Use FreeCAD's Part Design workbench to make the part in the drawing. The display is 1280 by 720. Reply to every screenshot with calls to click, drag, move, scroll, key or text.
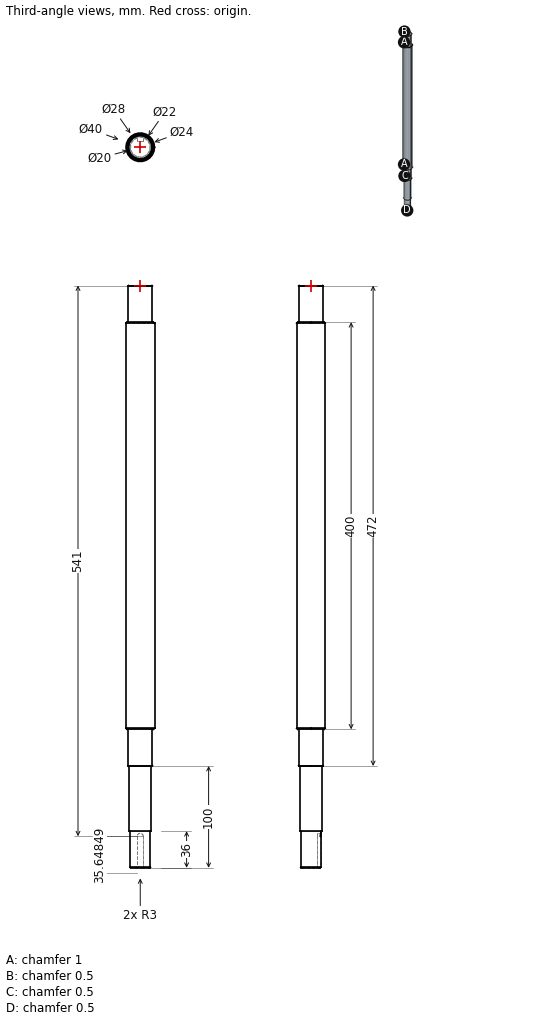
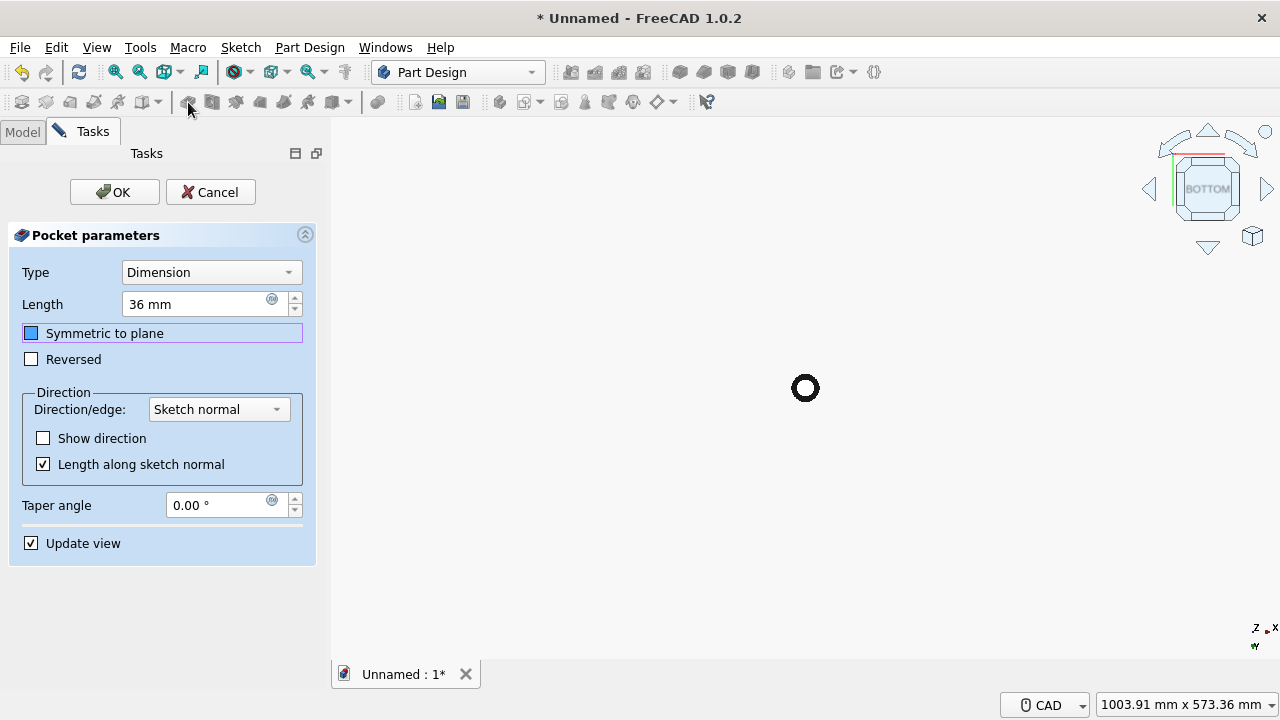
click(115, 192)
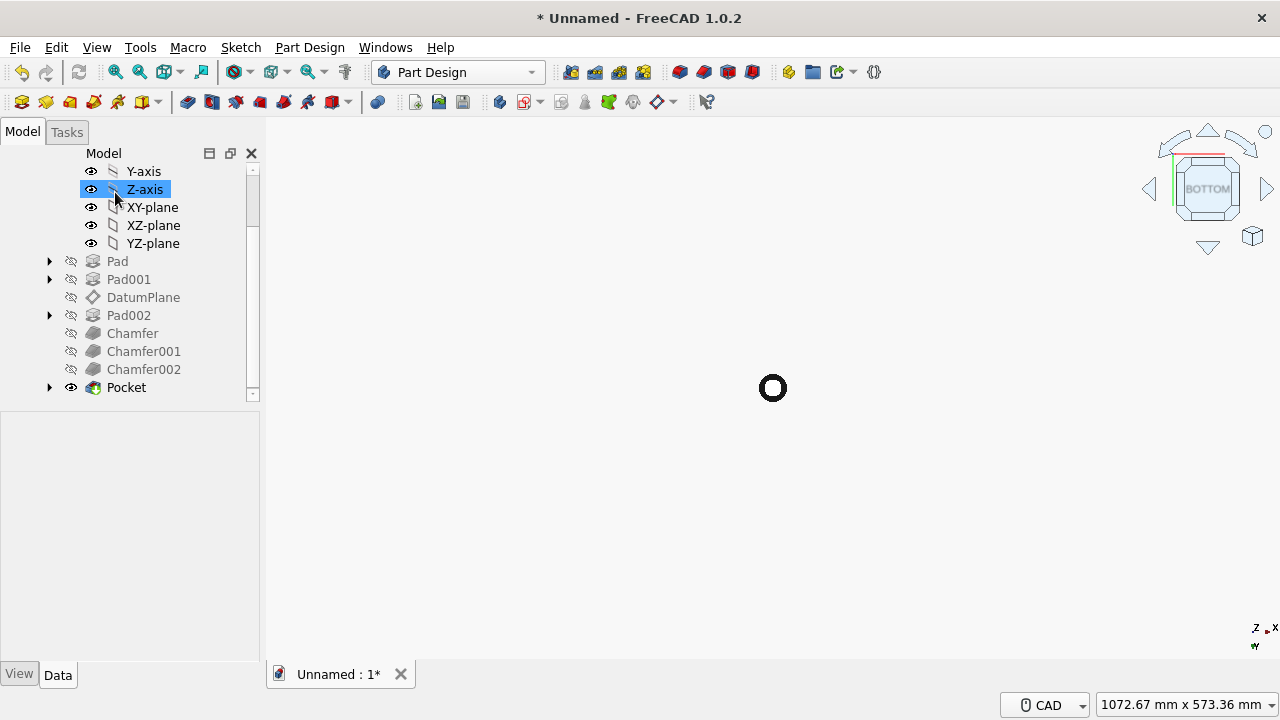
key(v)
key(f)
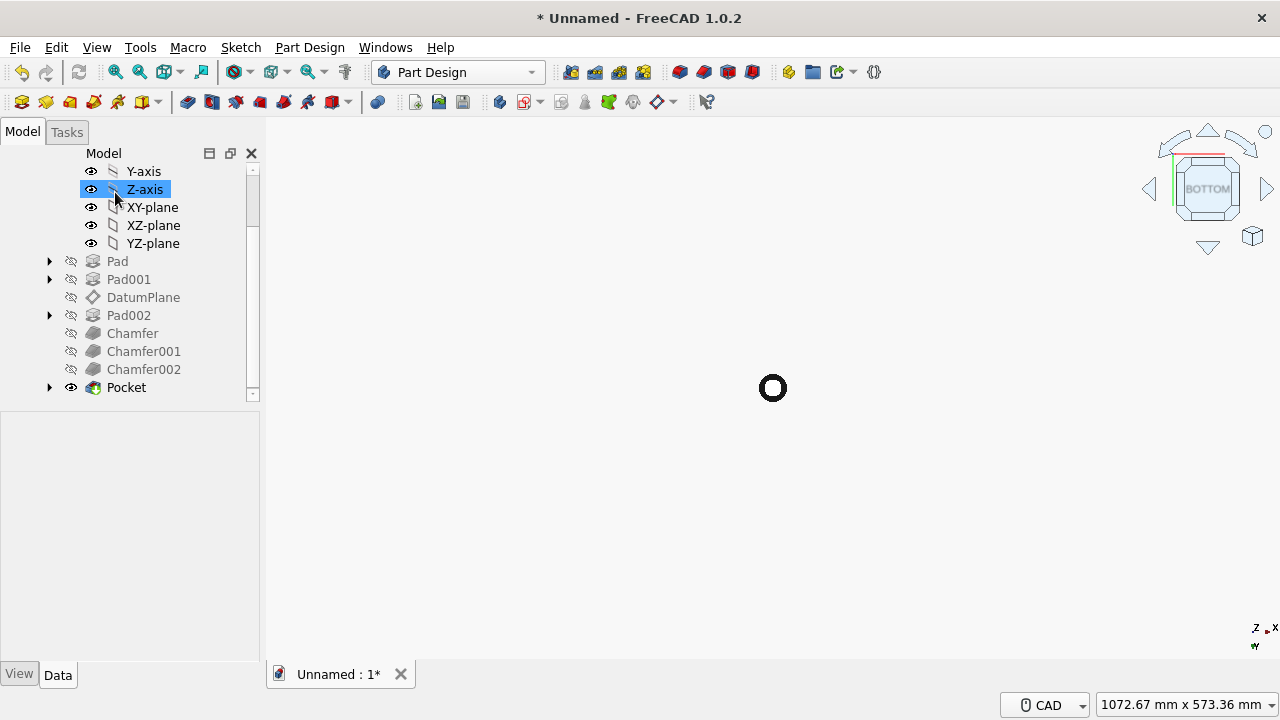
scroll(160, 275, down, 3)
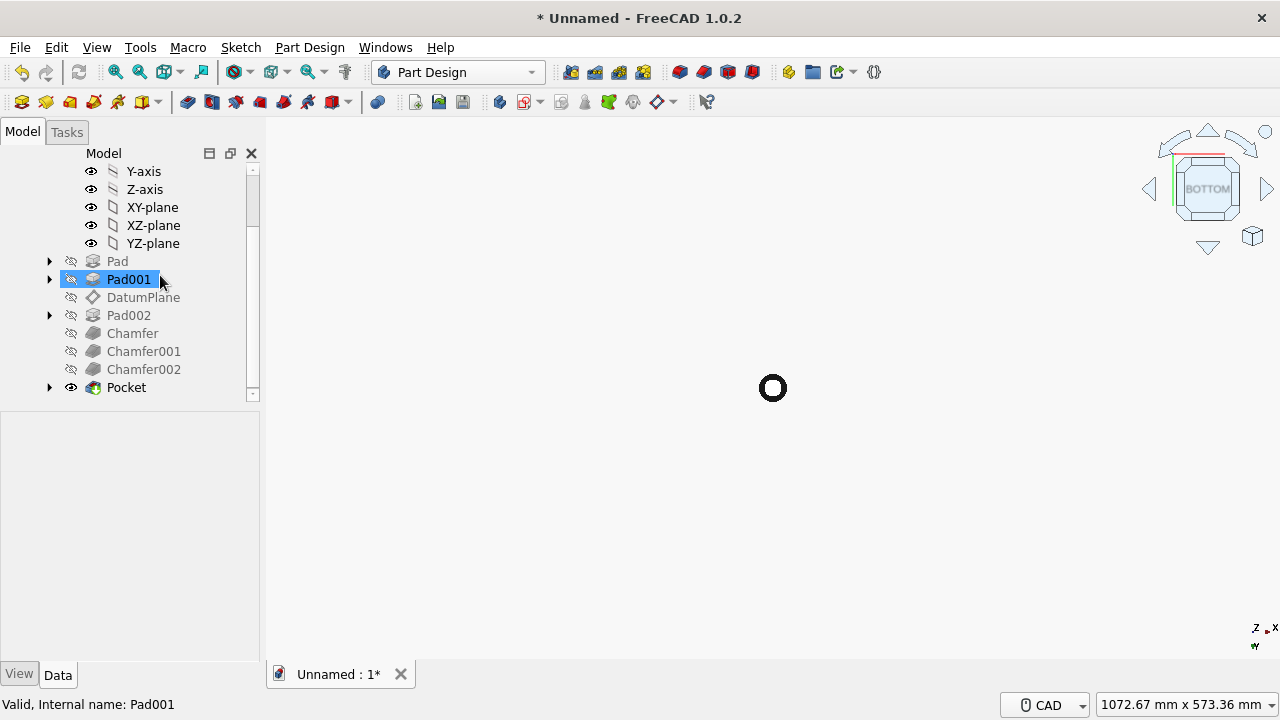
scroll(160, 275, up, 15)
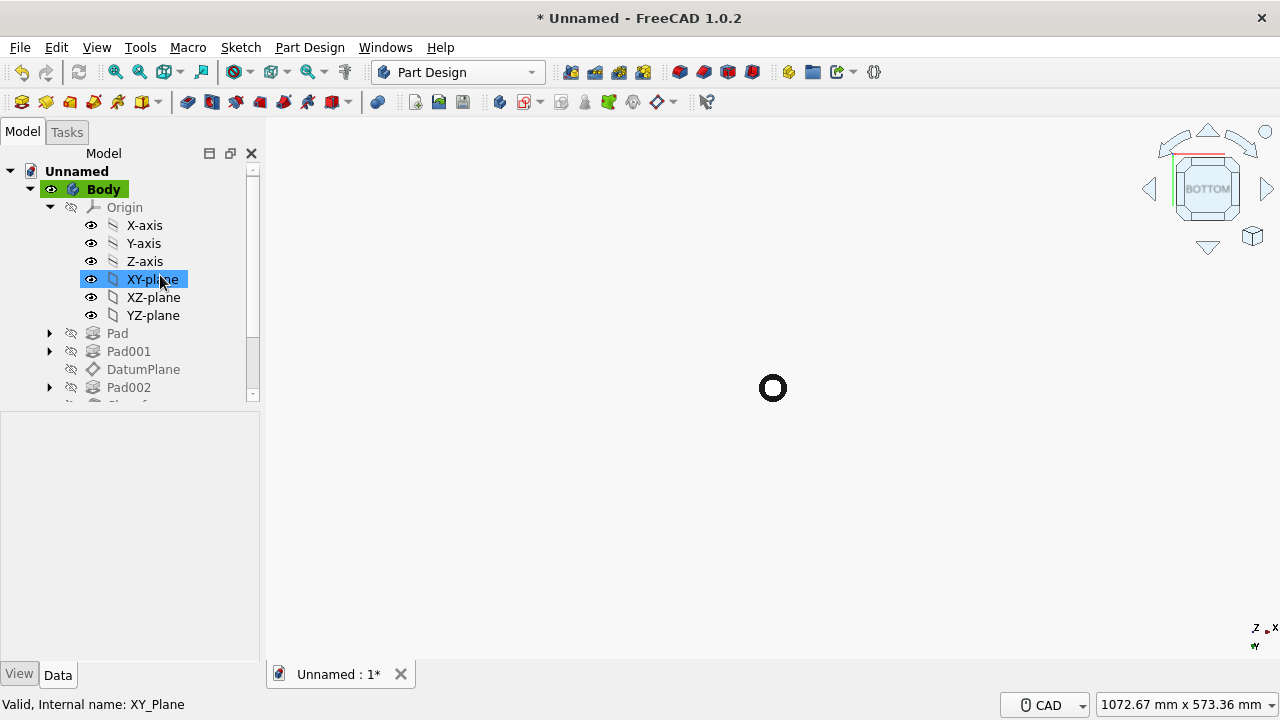
click(136, 297)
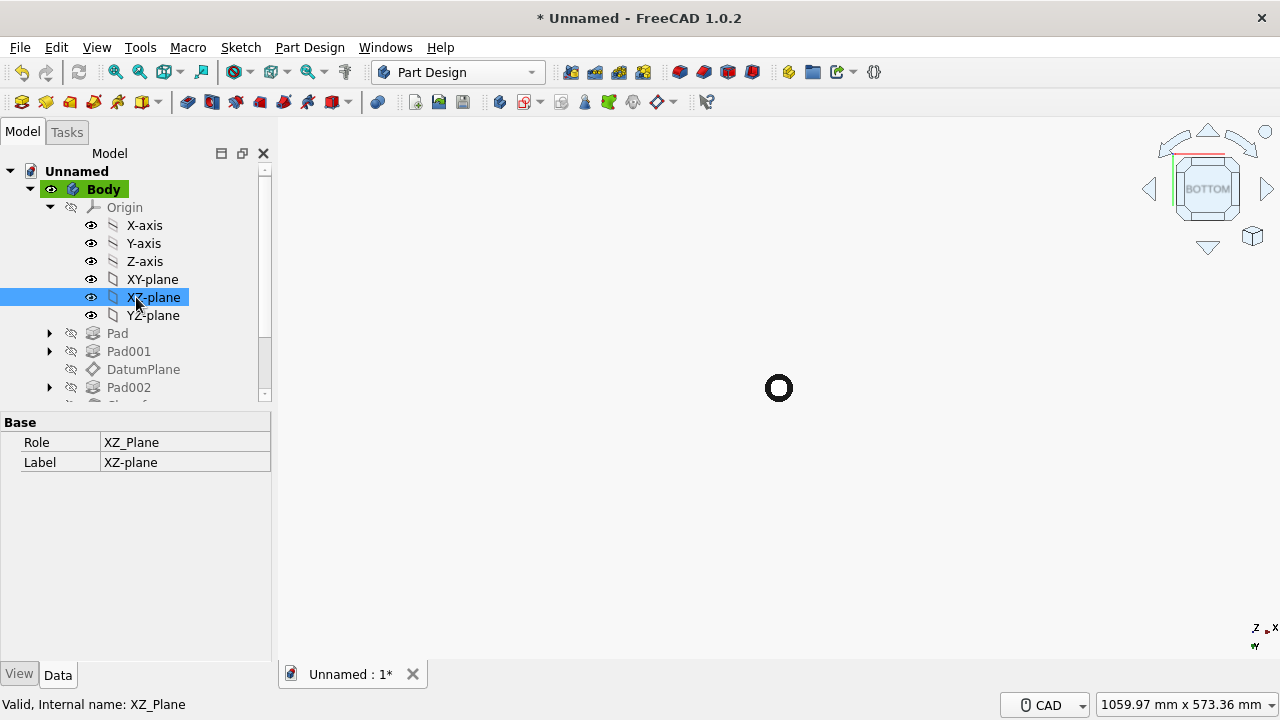
click(658, 102)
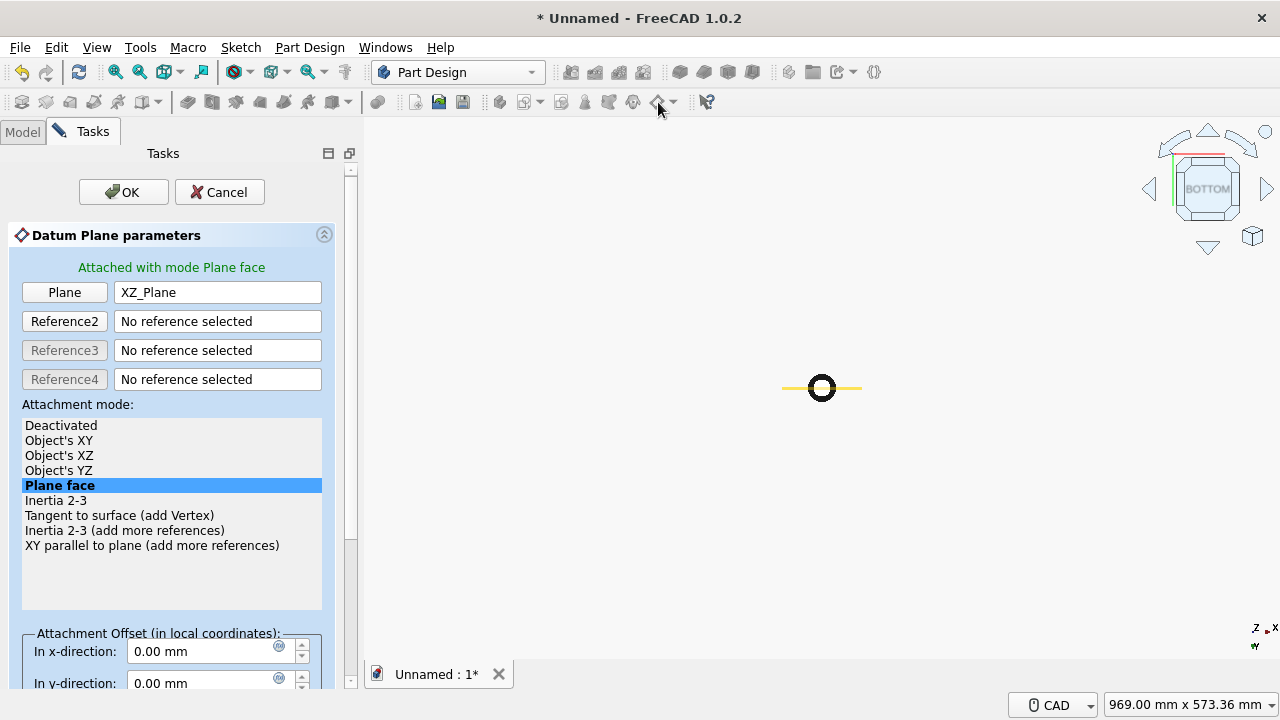
scroll(351, 426, down, 2)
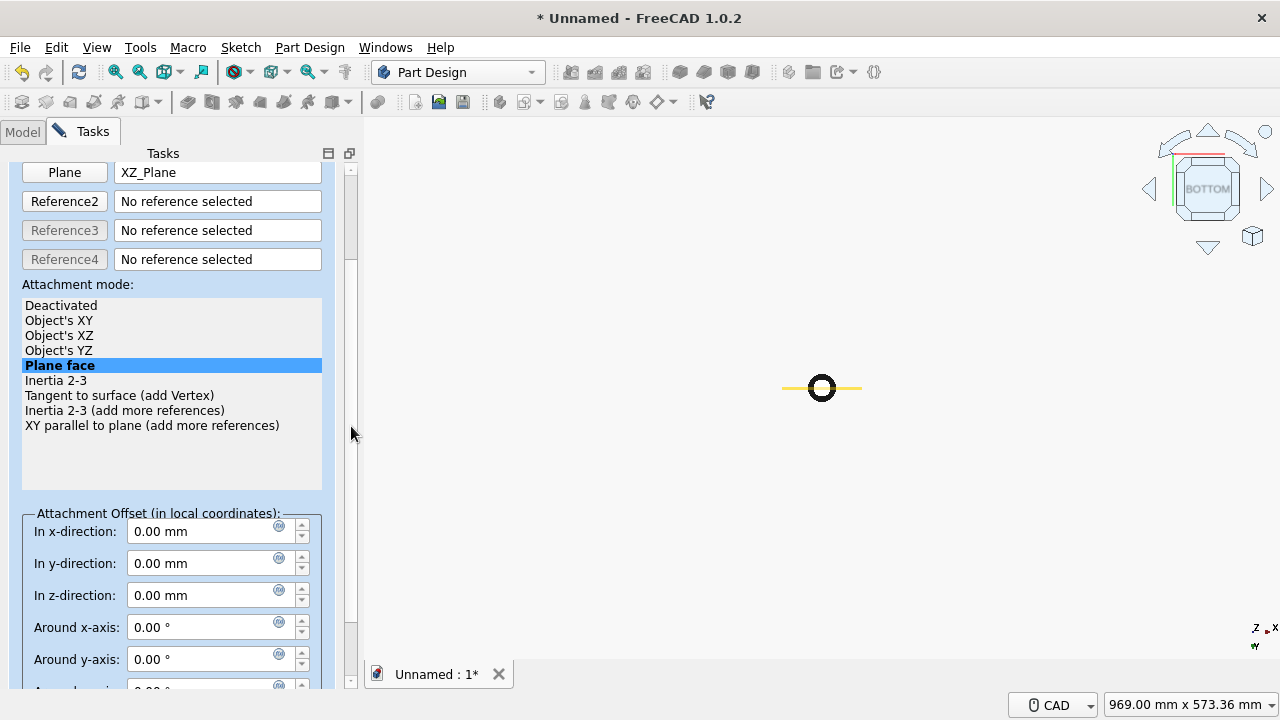
triple_click(210, 595)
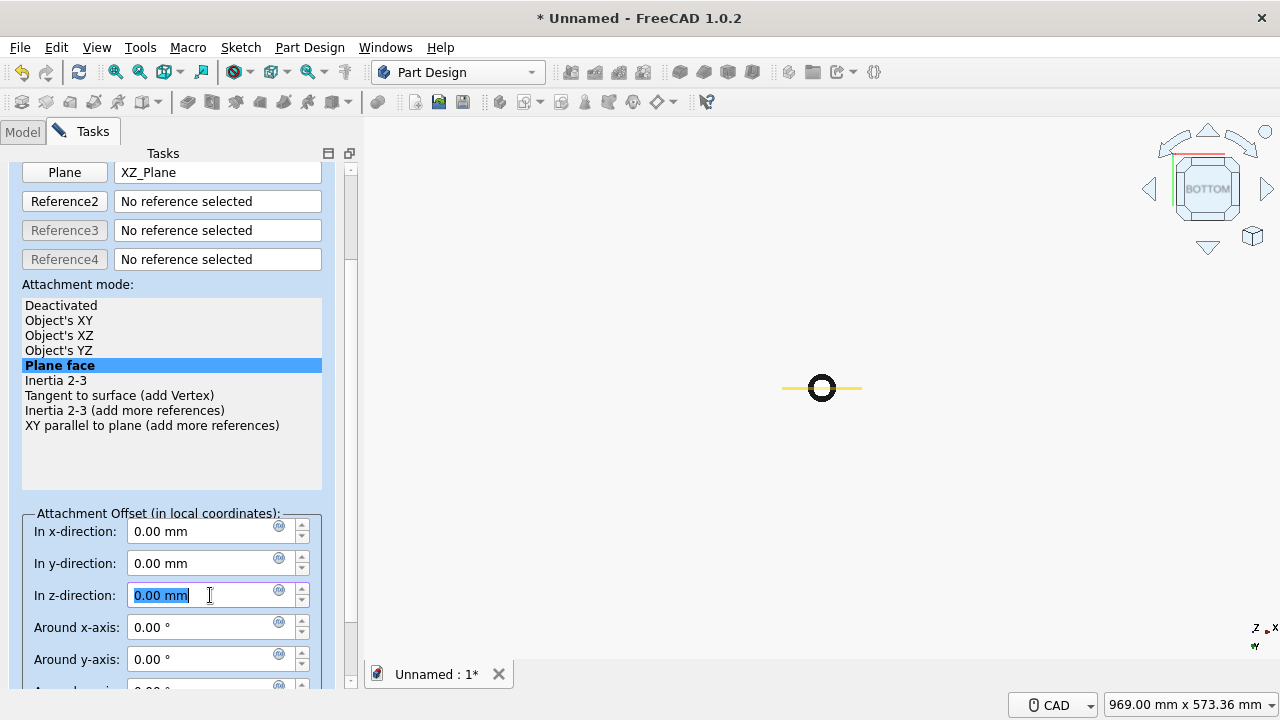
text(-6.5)
key(Tab)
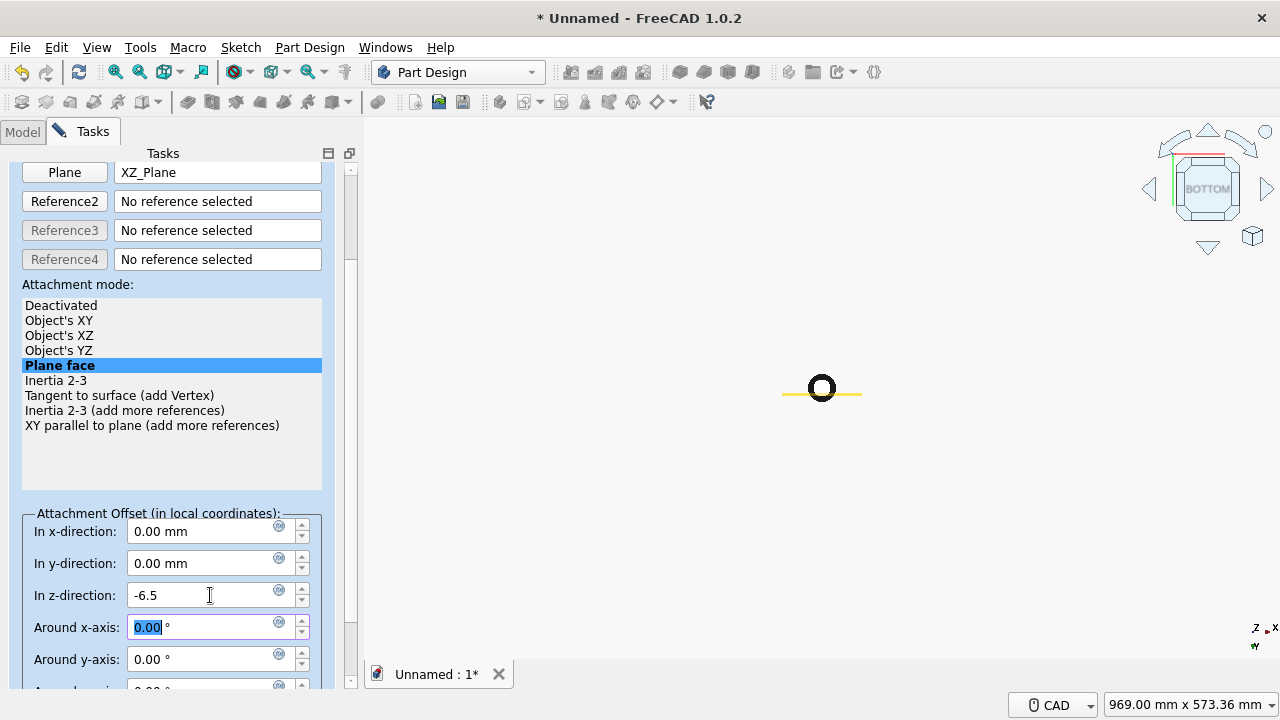
scroll(351, 426, up, 3)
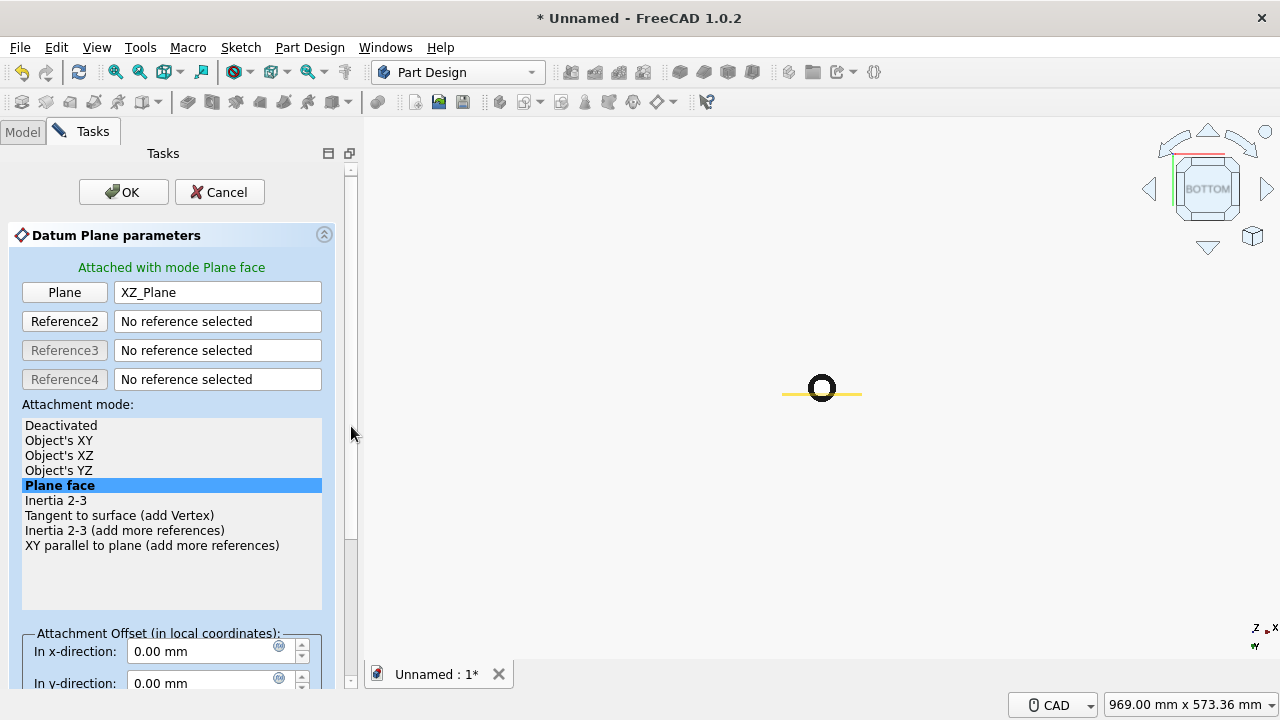
click(124, 192)